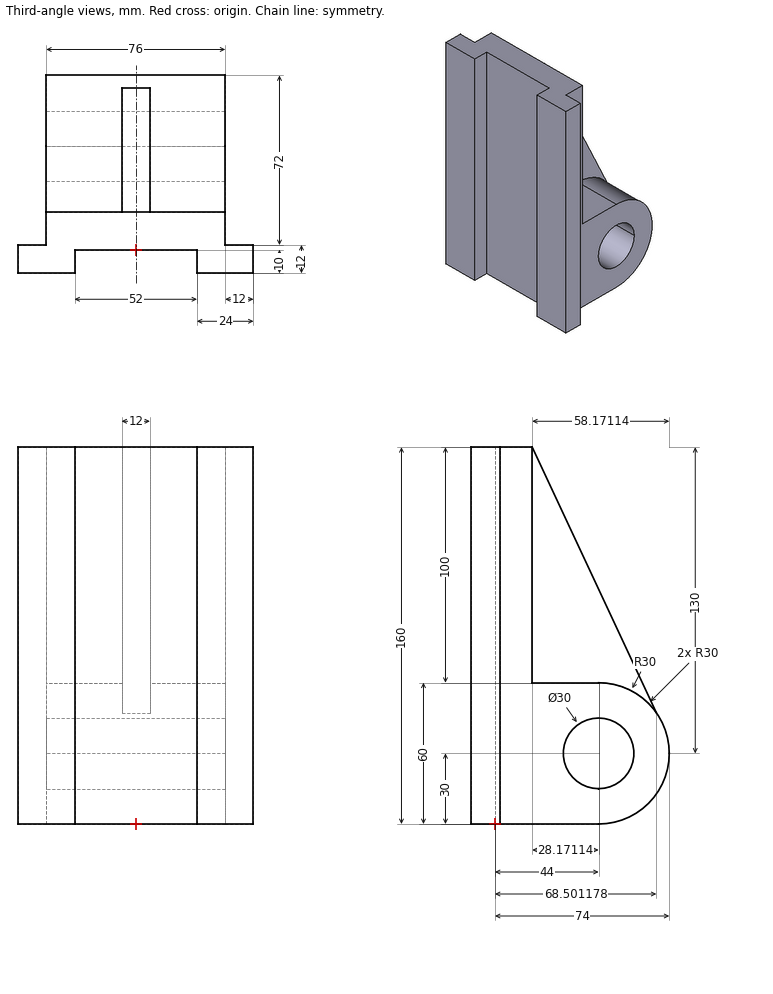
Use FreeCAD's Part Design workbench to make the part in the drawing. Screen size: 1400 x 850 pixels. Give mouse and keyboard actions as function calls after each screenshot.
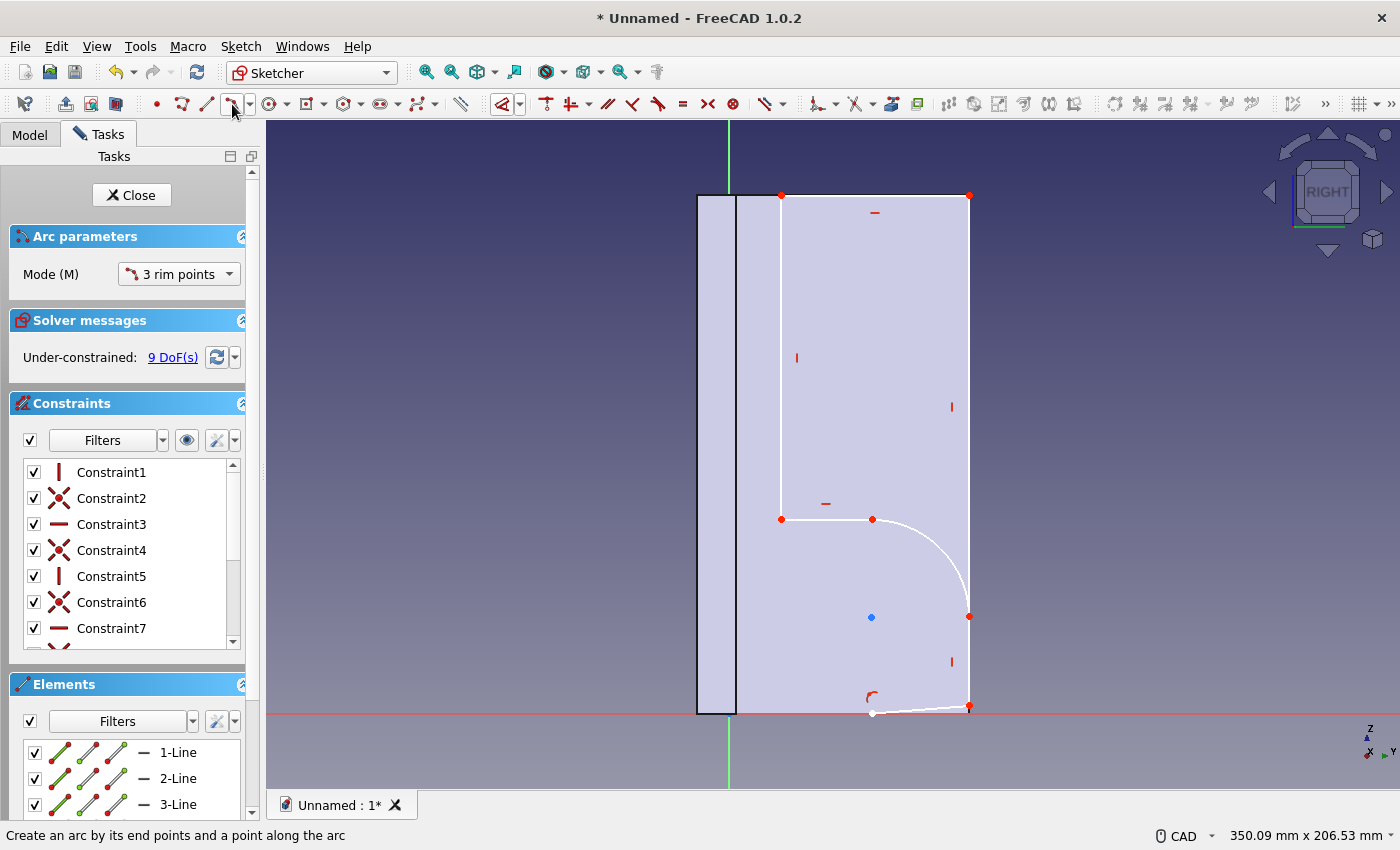
click(969, 617)
click(872, 714)
click(941, 685)
key(Escape)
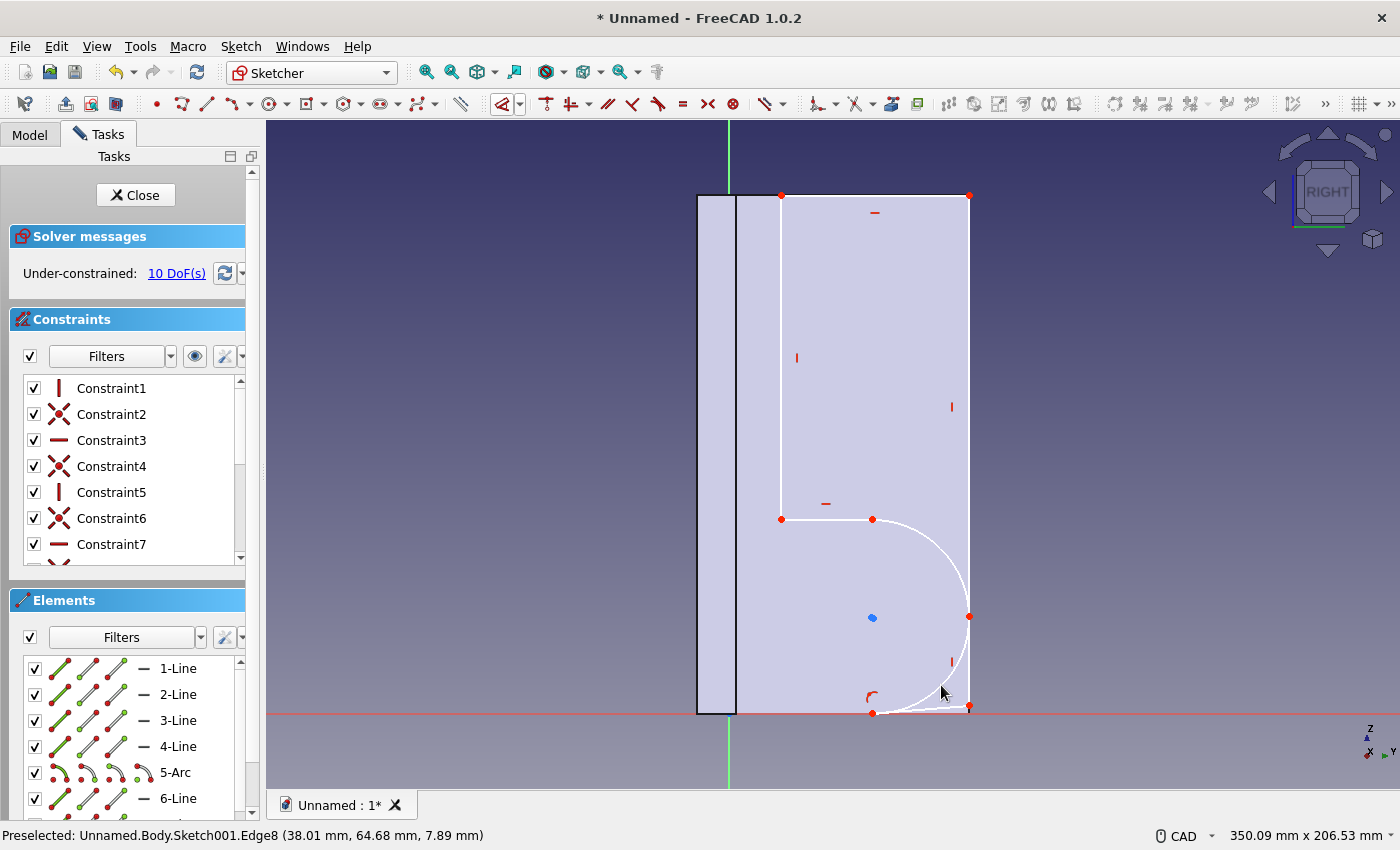
click(969, 491)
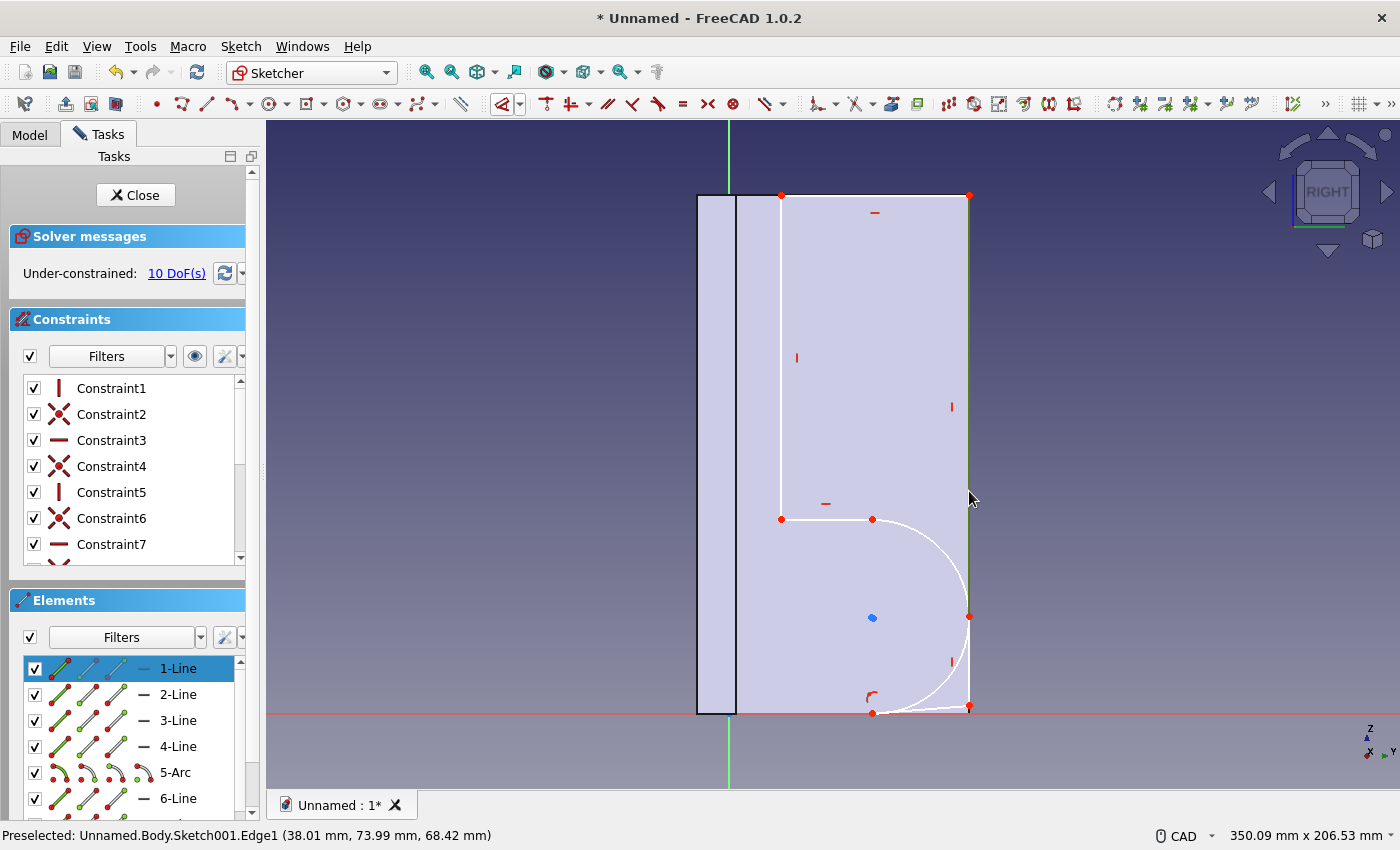
scroll(958, 573, up, 2)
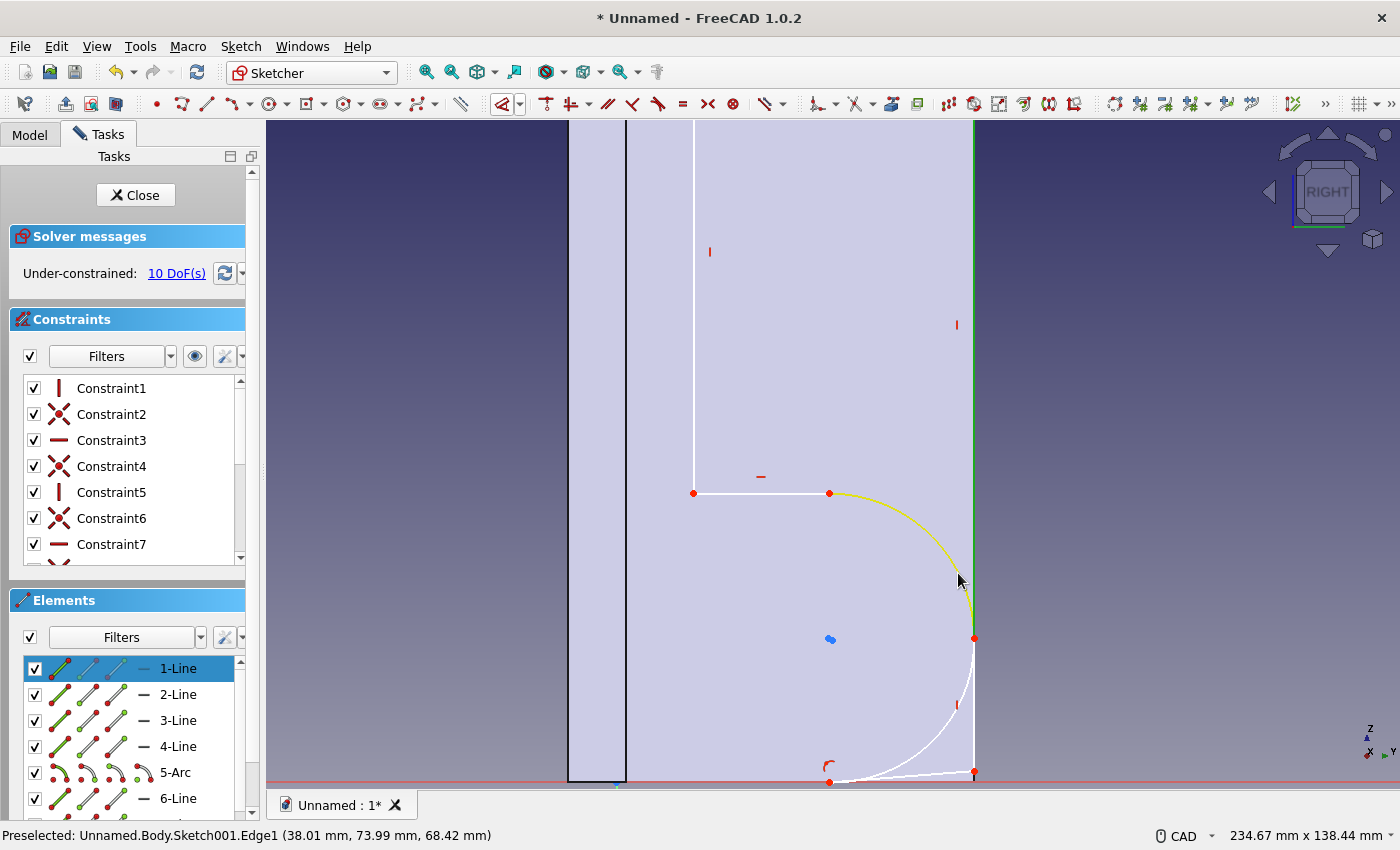
click(958, 573)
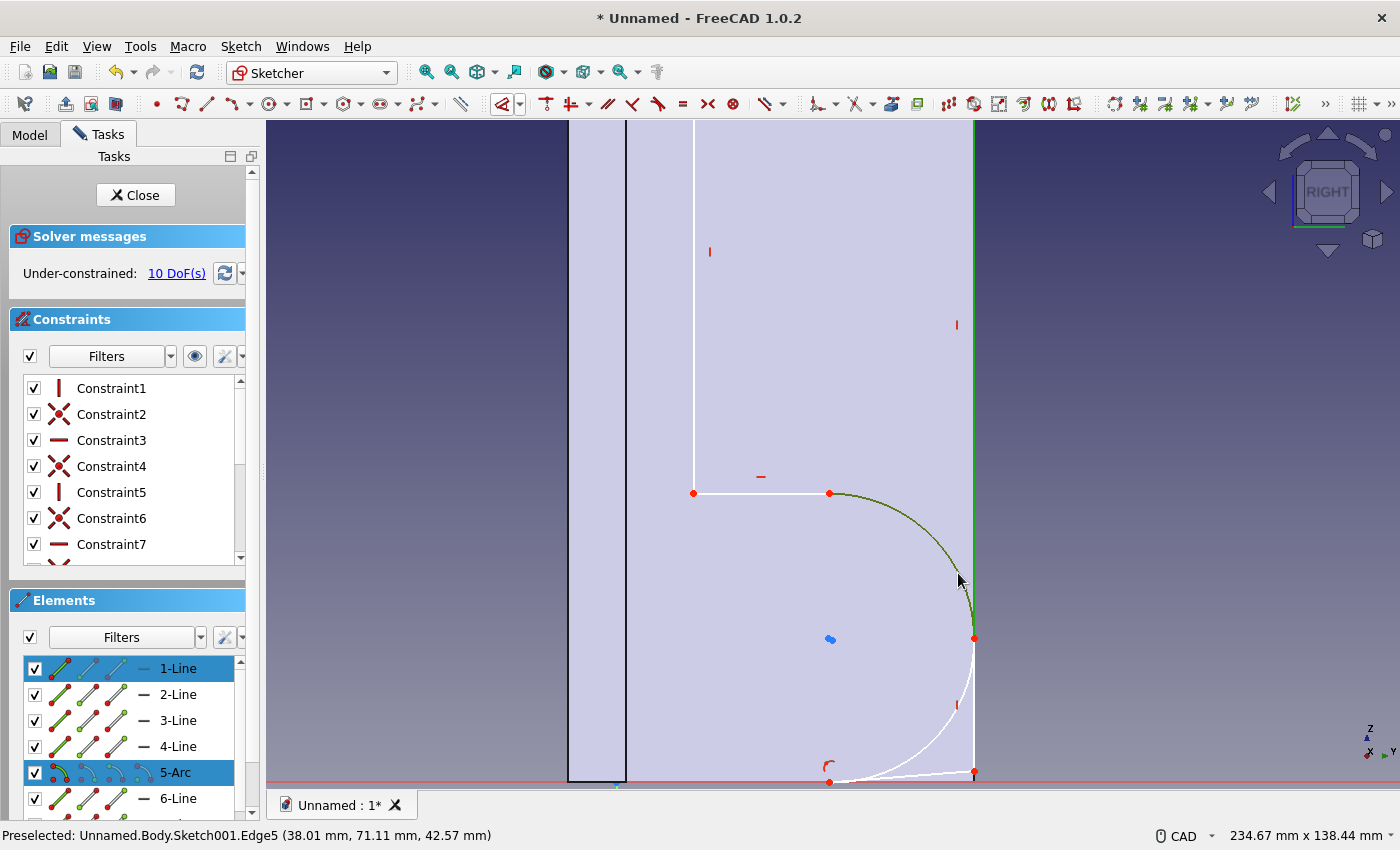
click(658, 104)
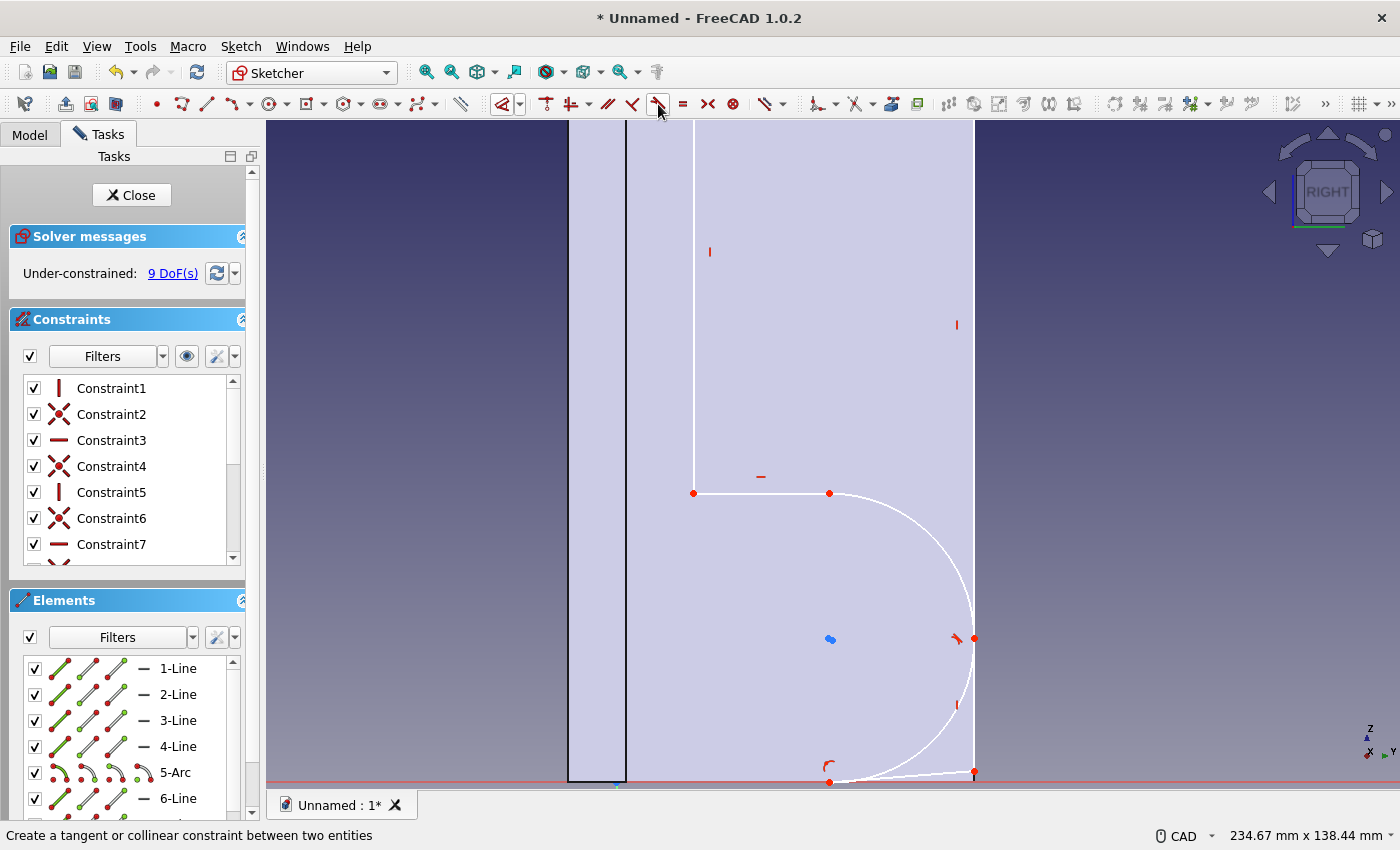
click(974, 450)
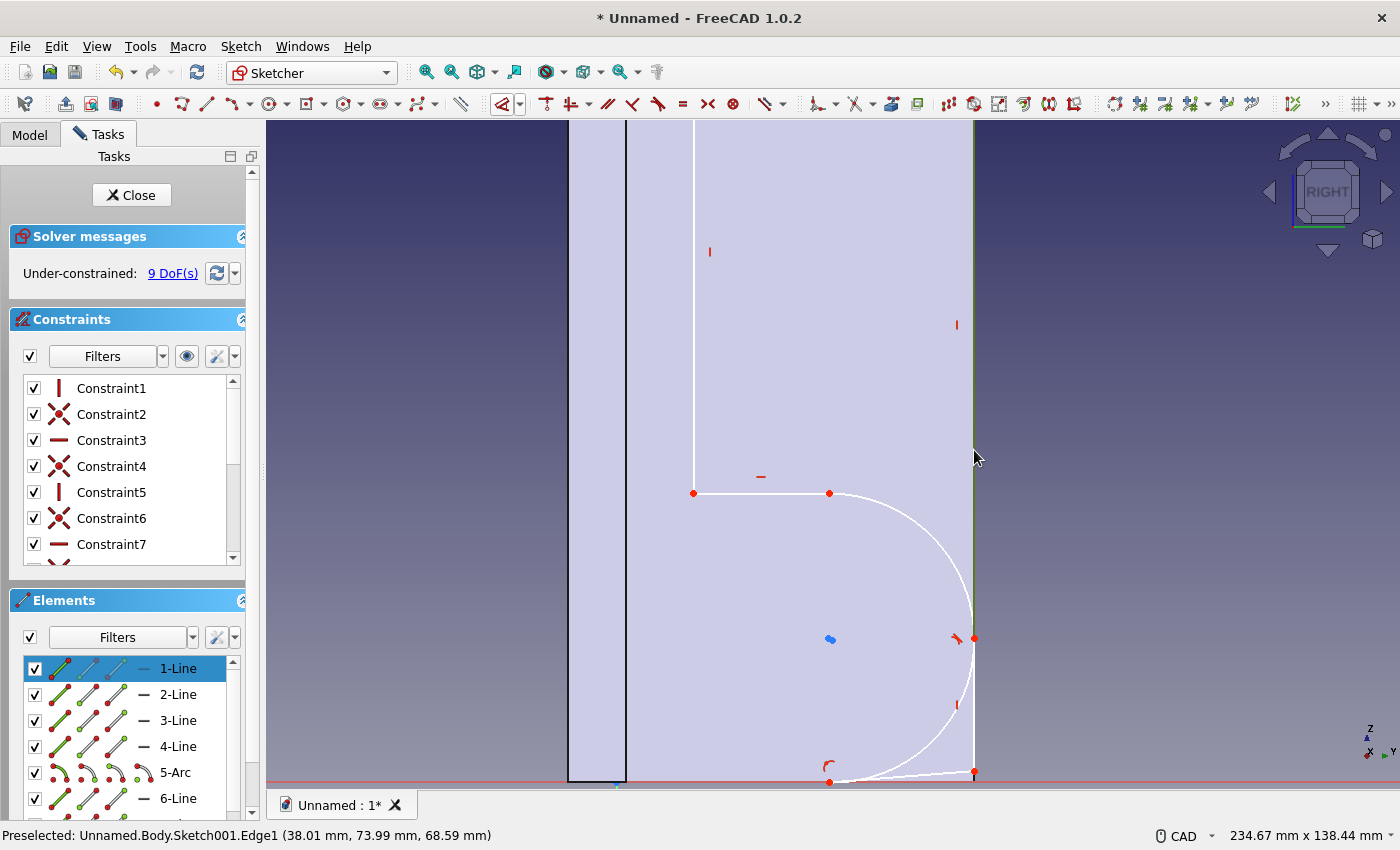
click(932, 741)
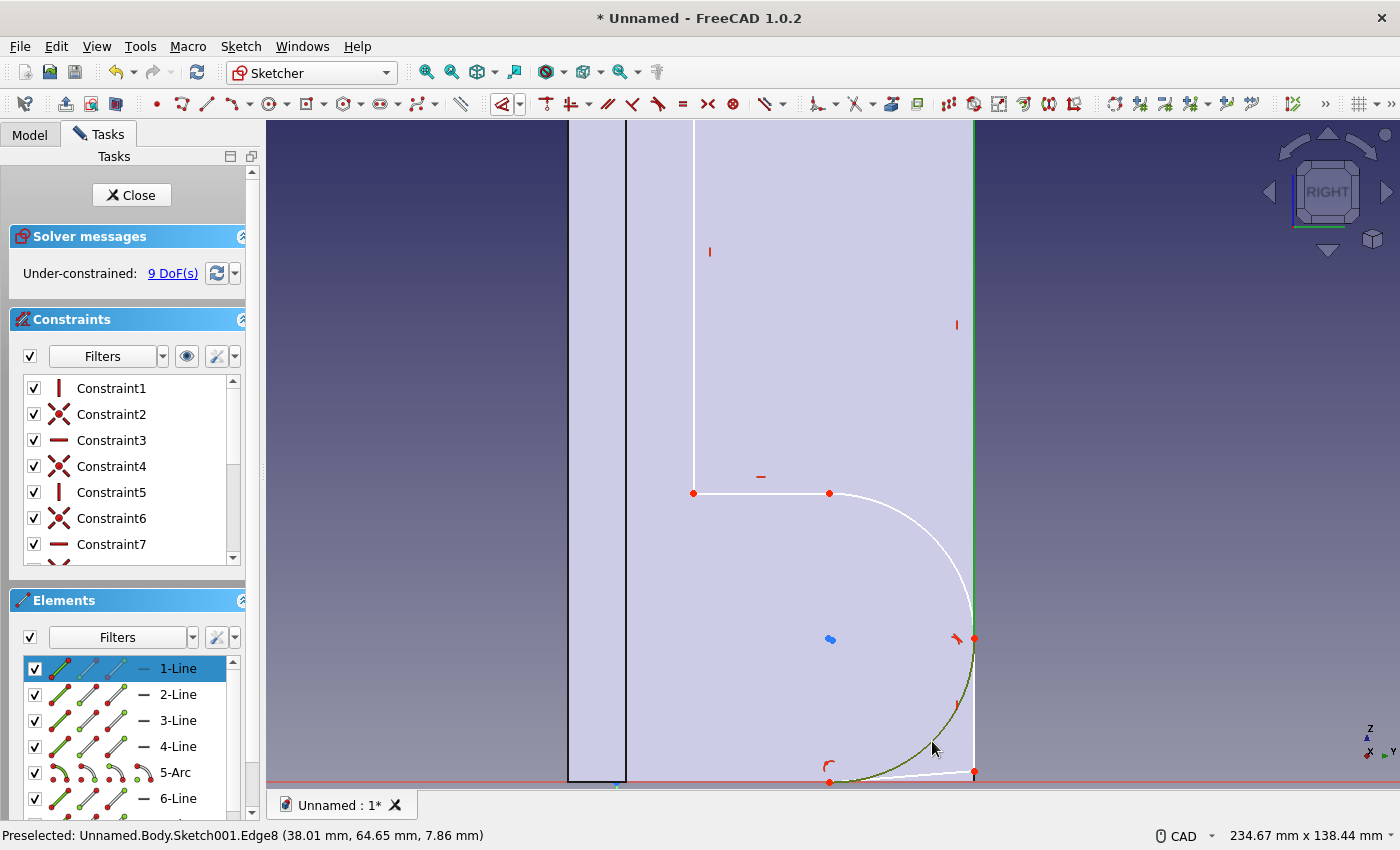
key(t)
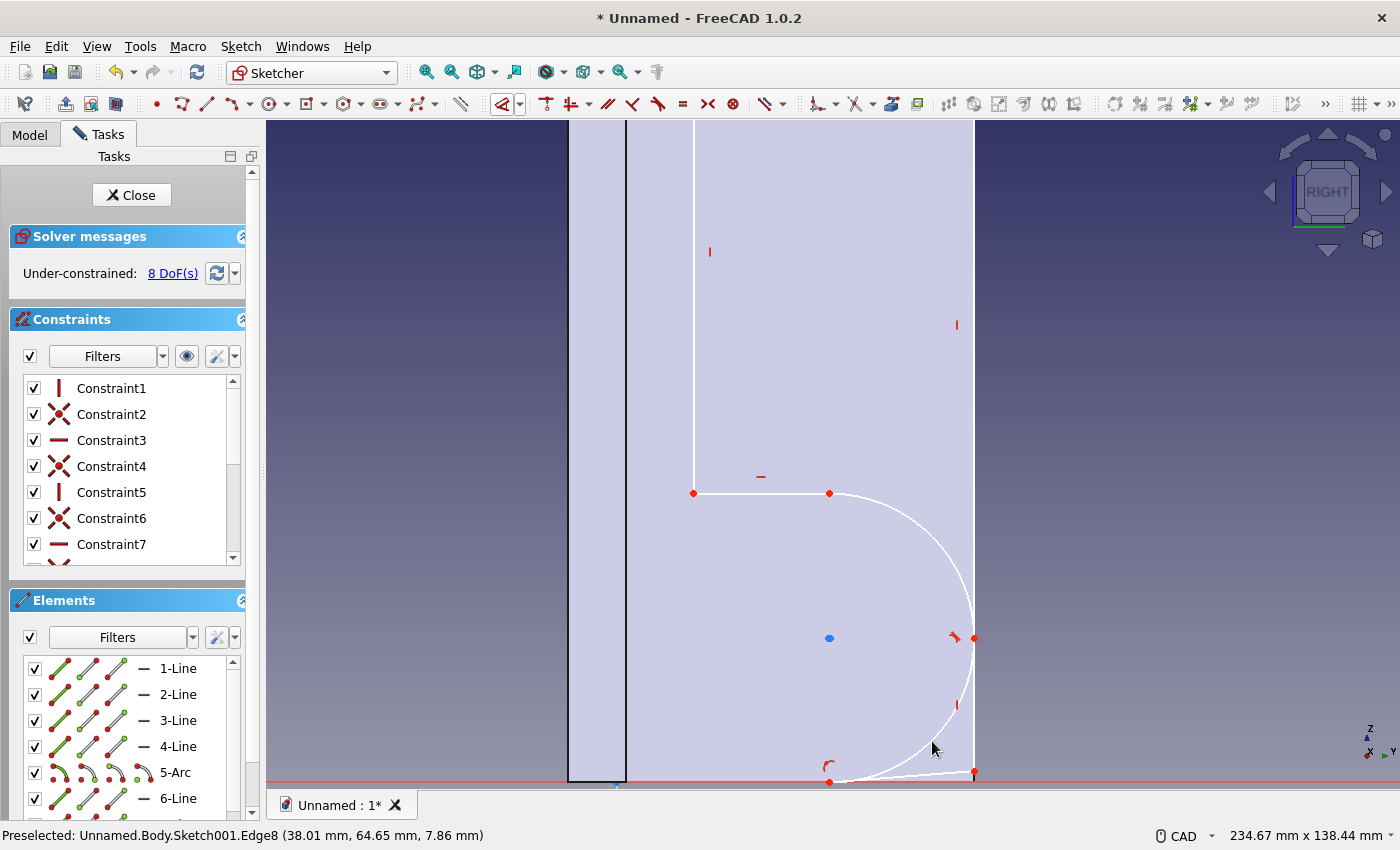
click(734, 494)